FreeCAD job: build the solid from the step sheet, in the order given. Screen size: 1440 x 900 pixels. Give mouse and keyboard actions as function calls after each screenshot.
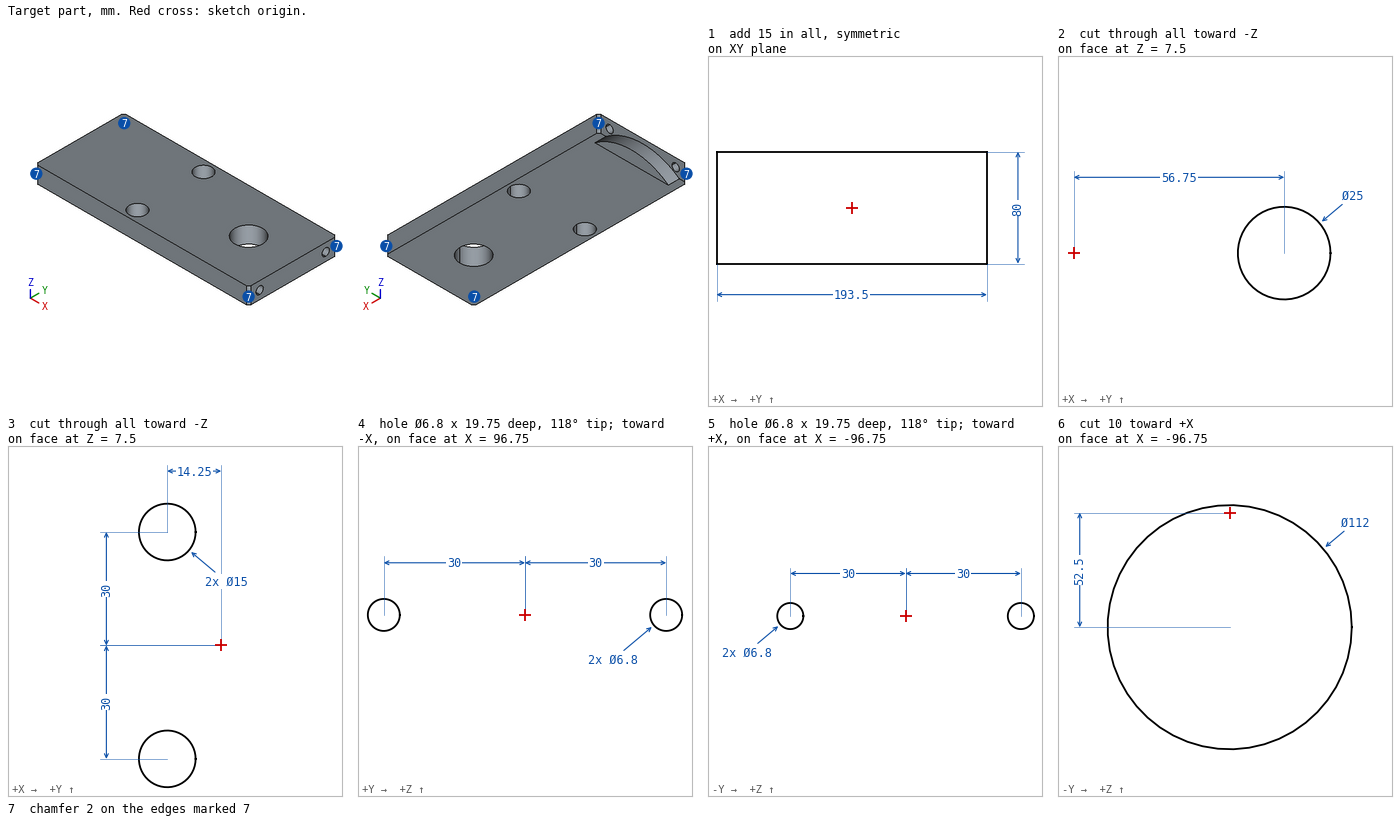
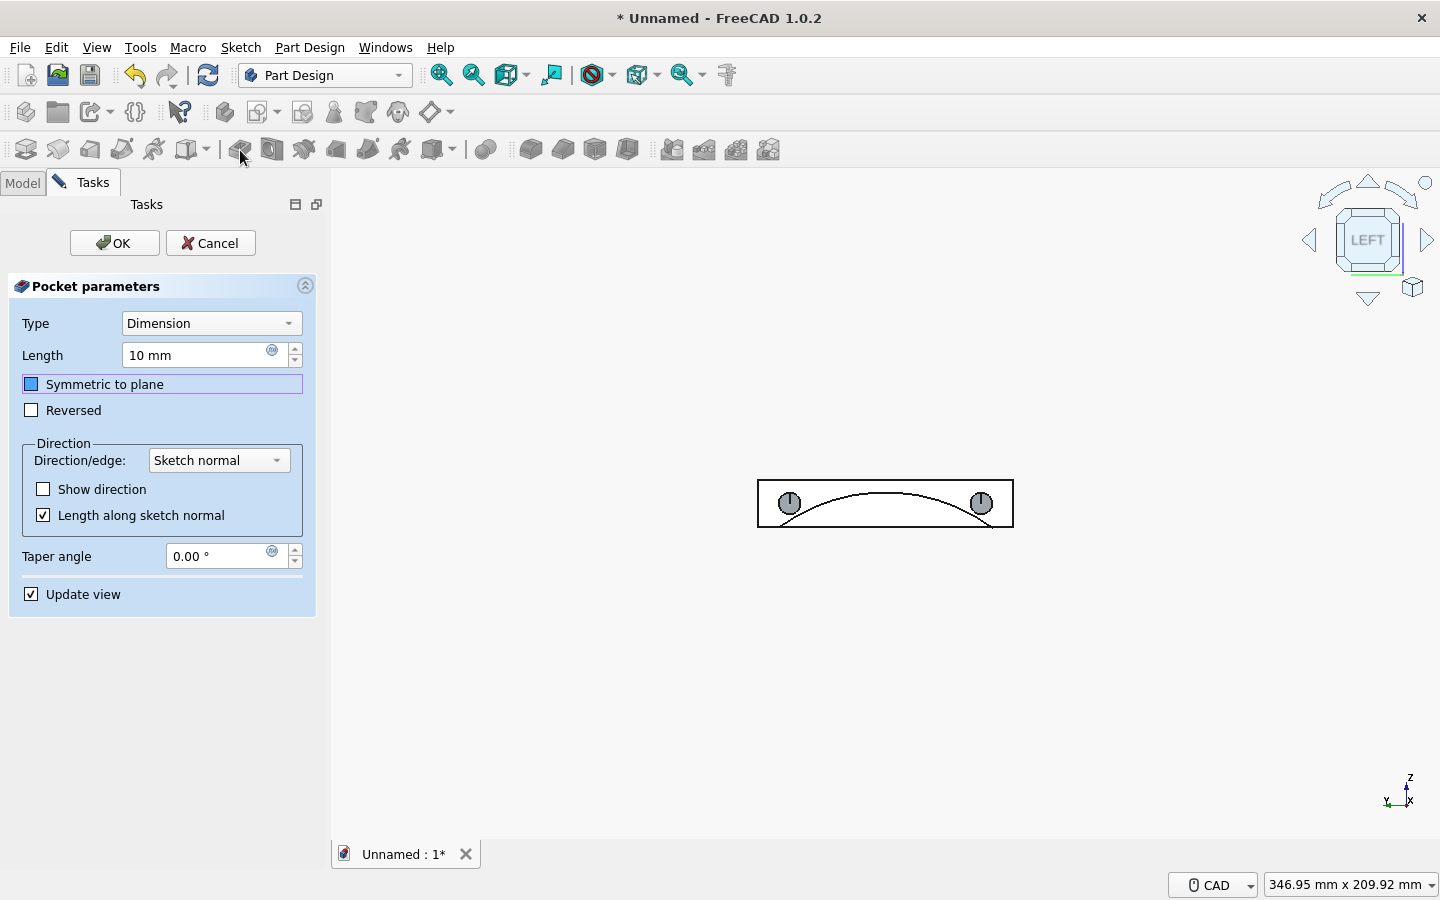
click(115, 243)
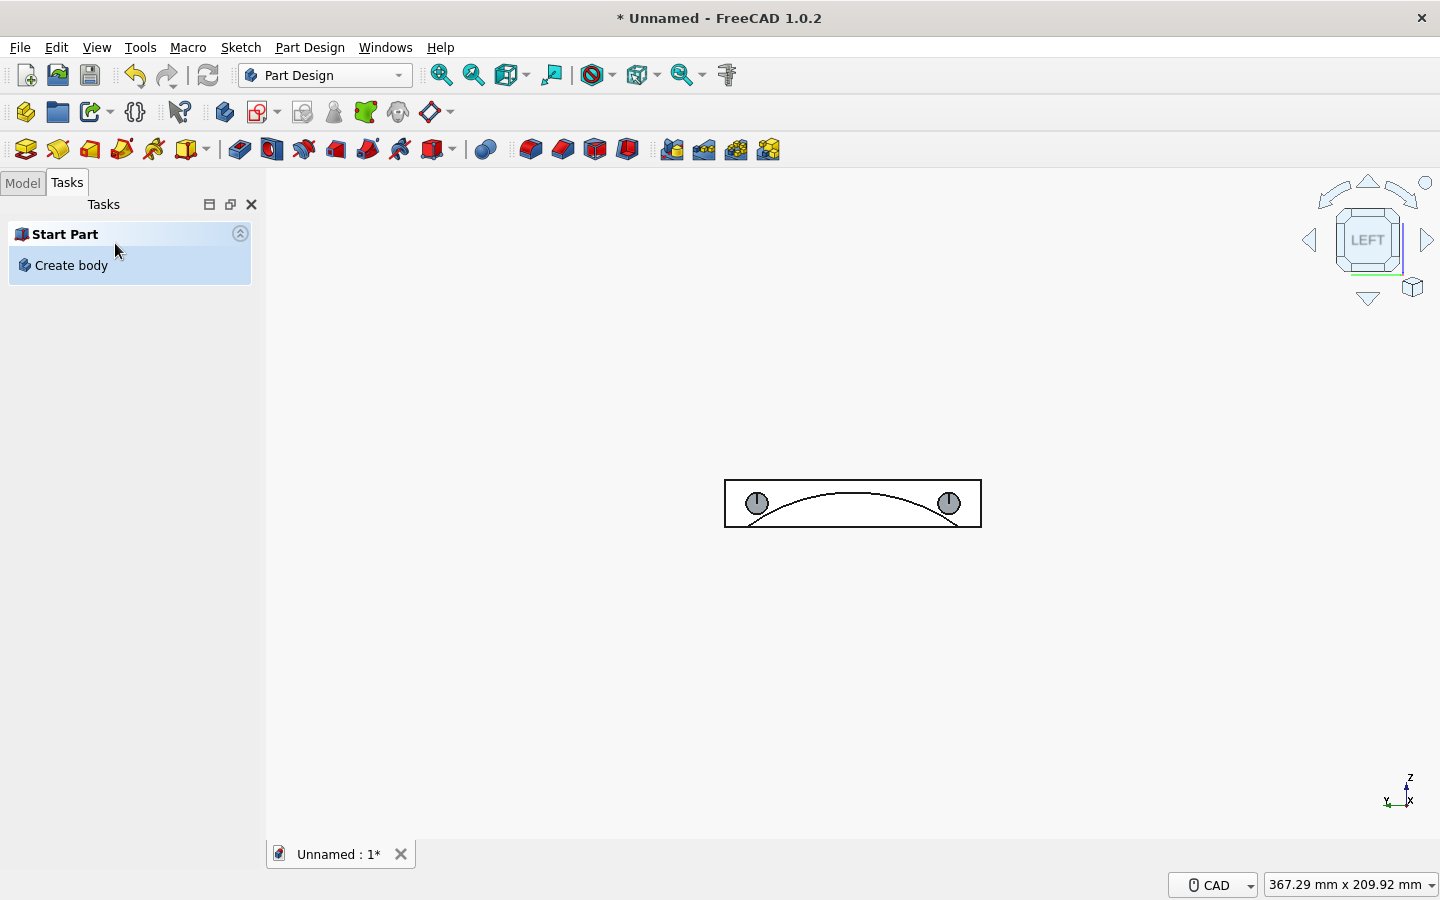
click(442, 76)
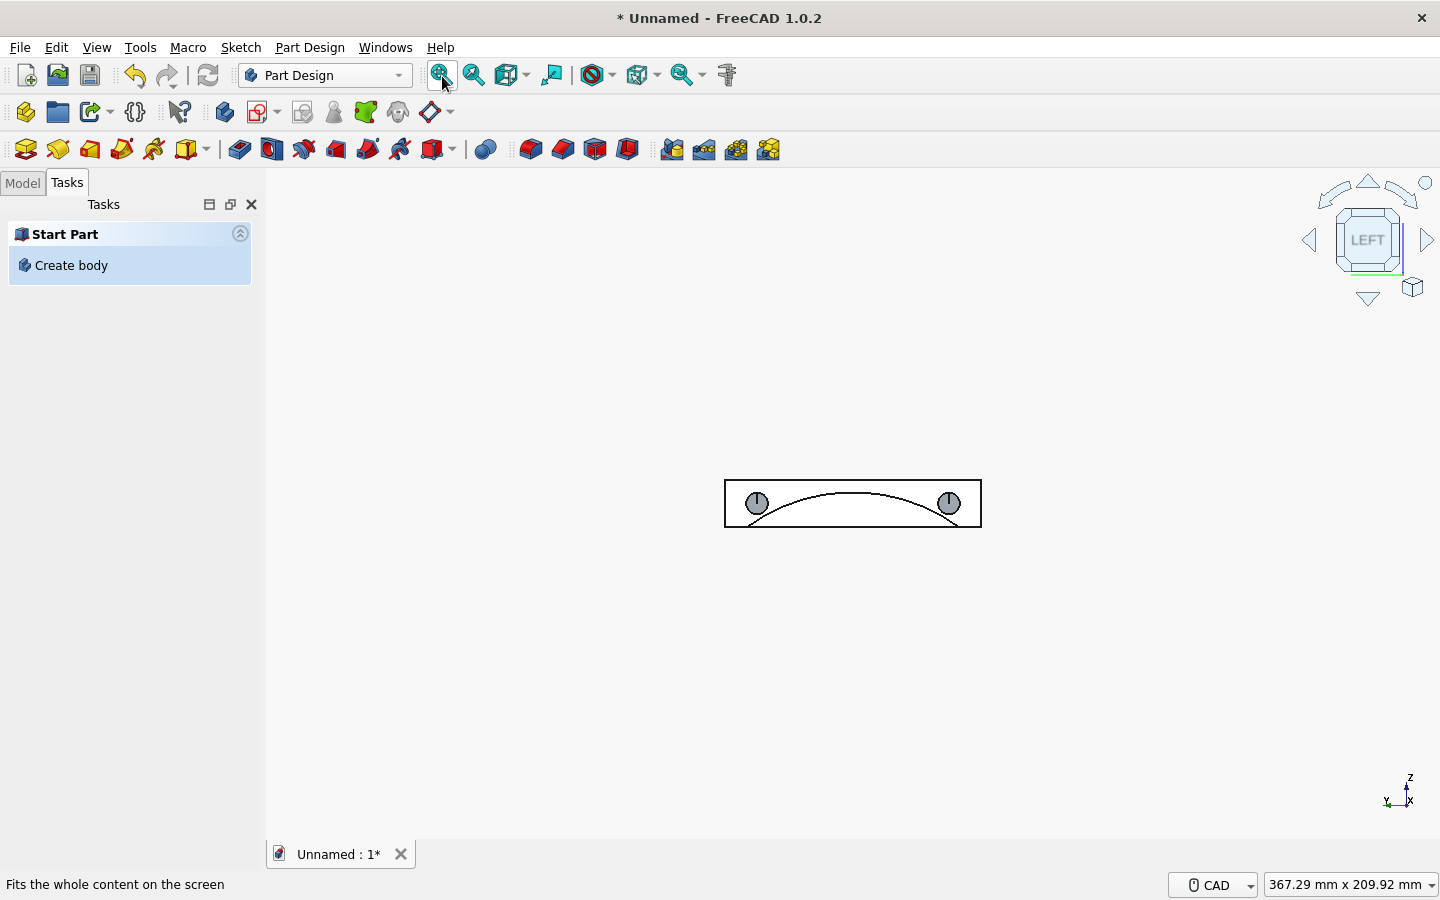
click(981, 502)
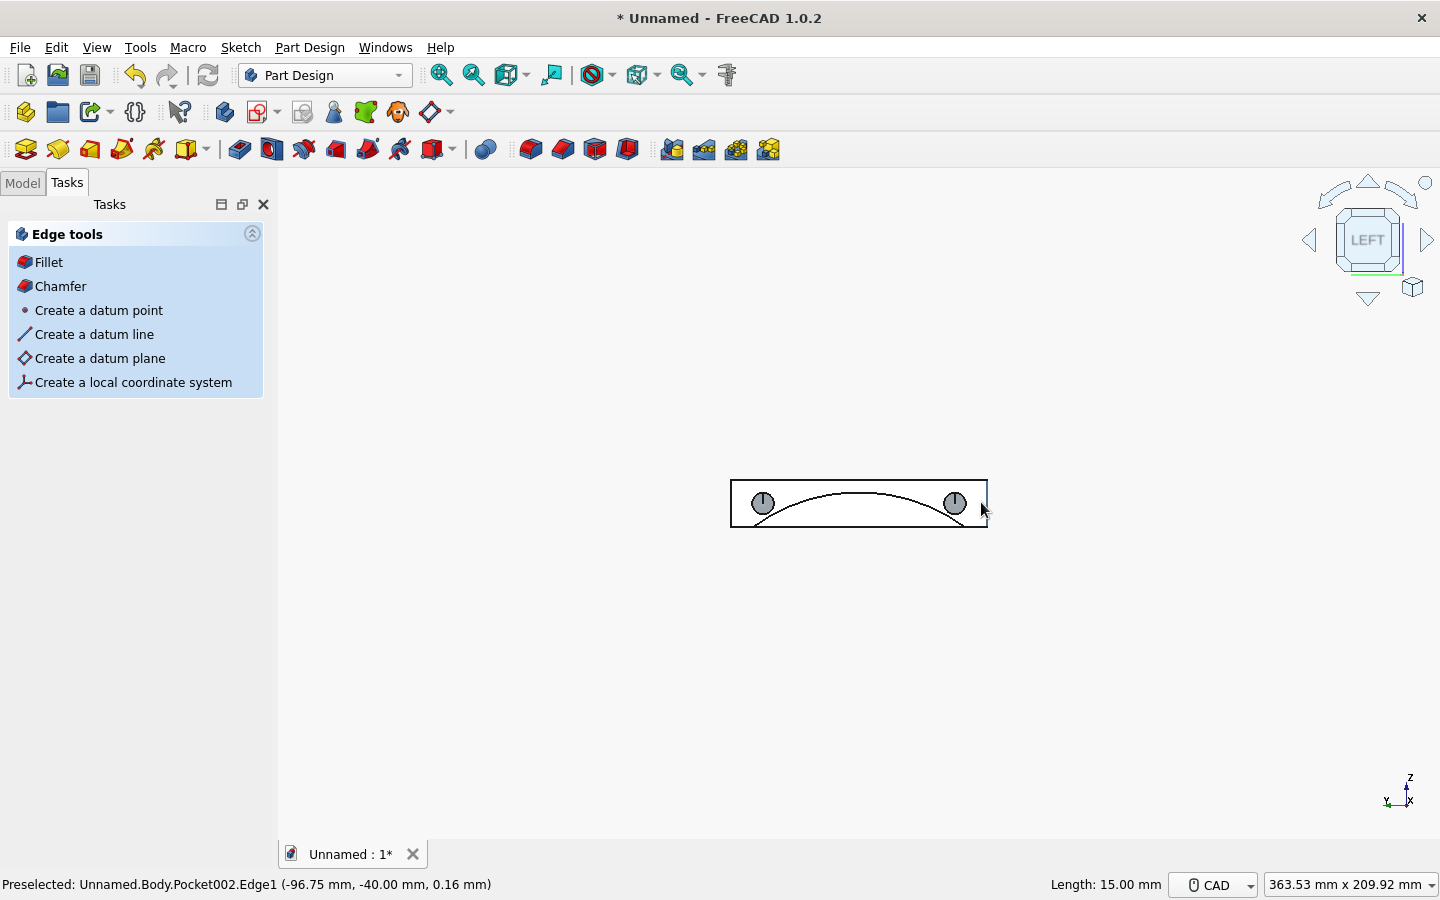
click(731, 502, ctrl)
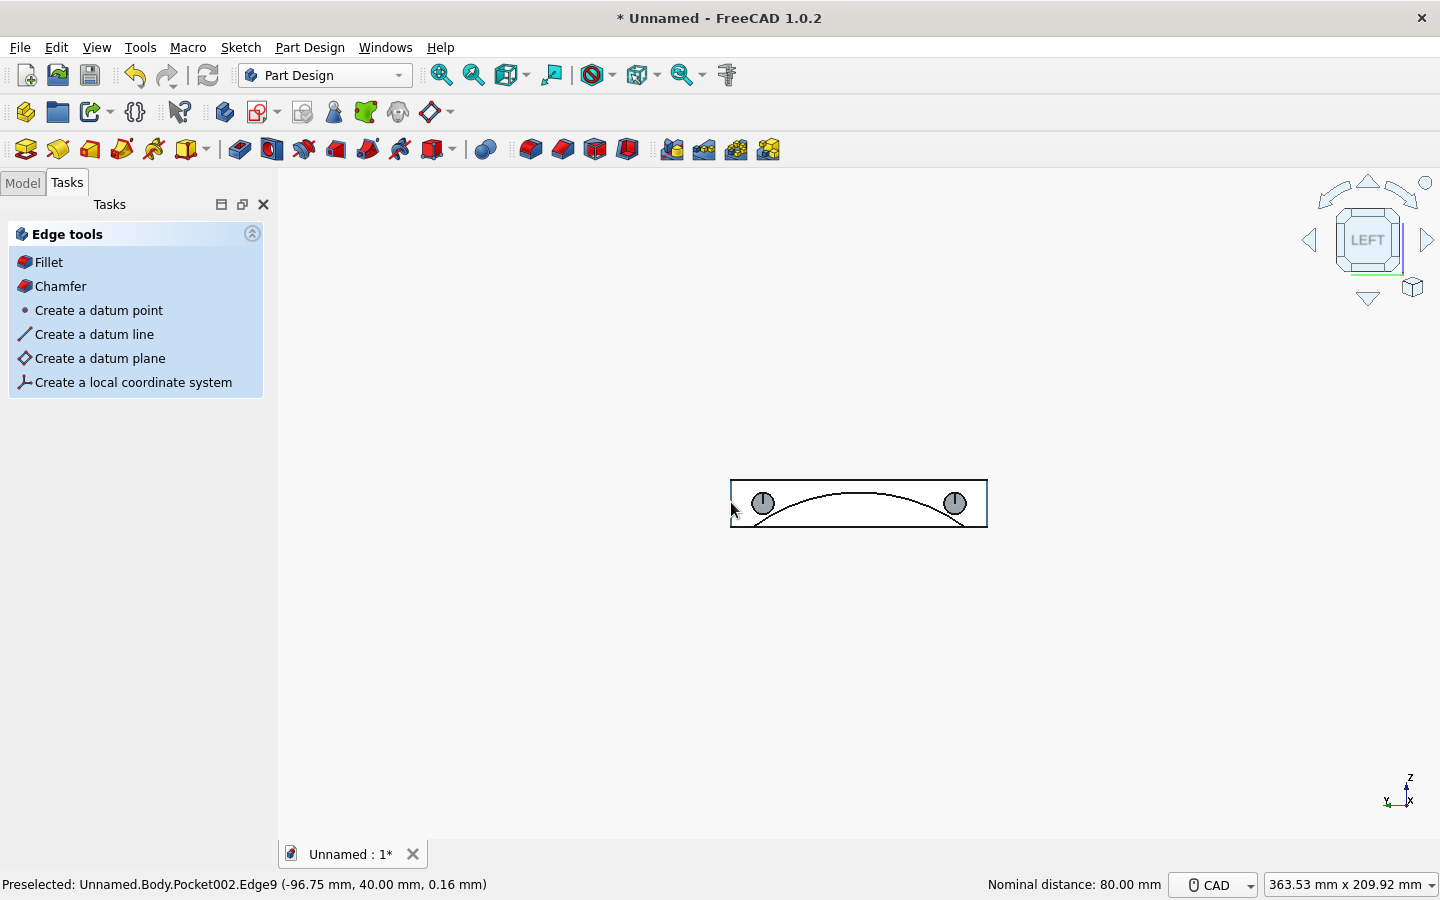
key(0)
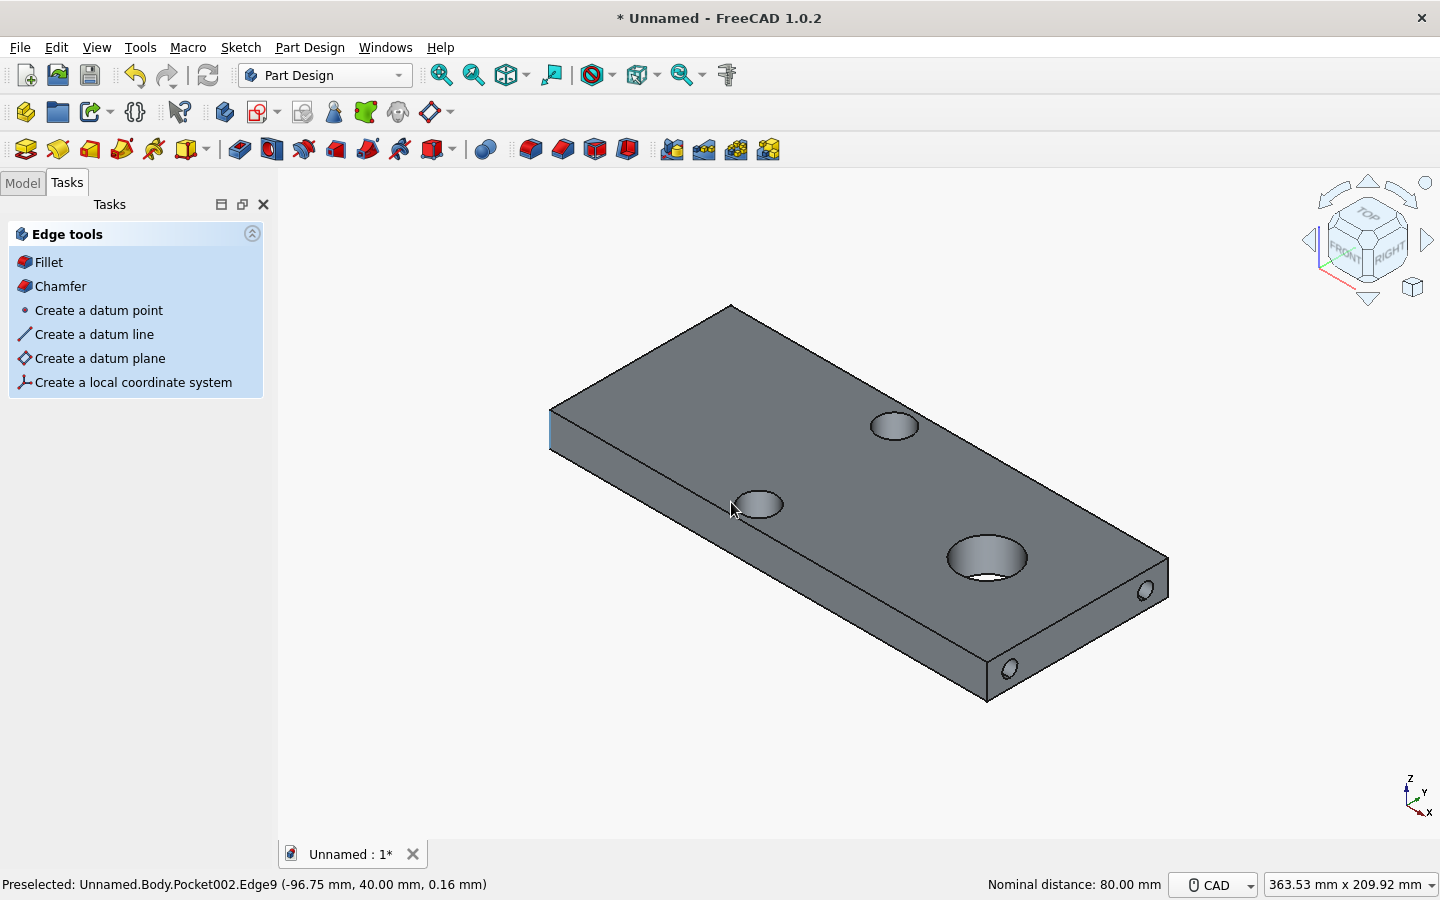
click(987, 681, ctrl)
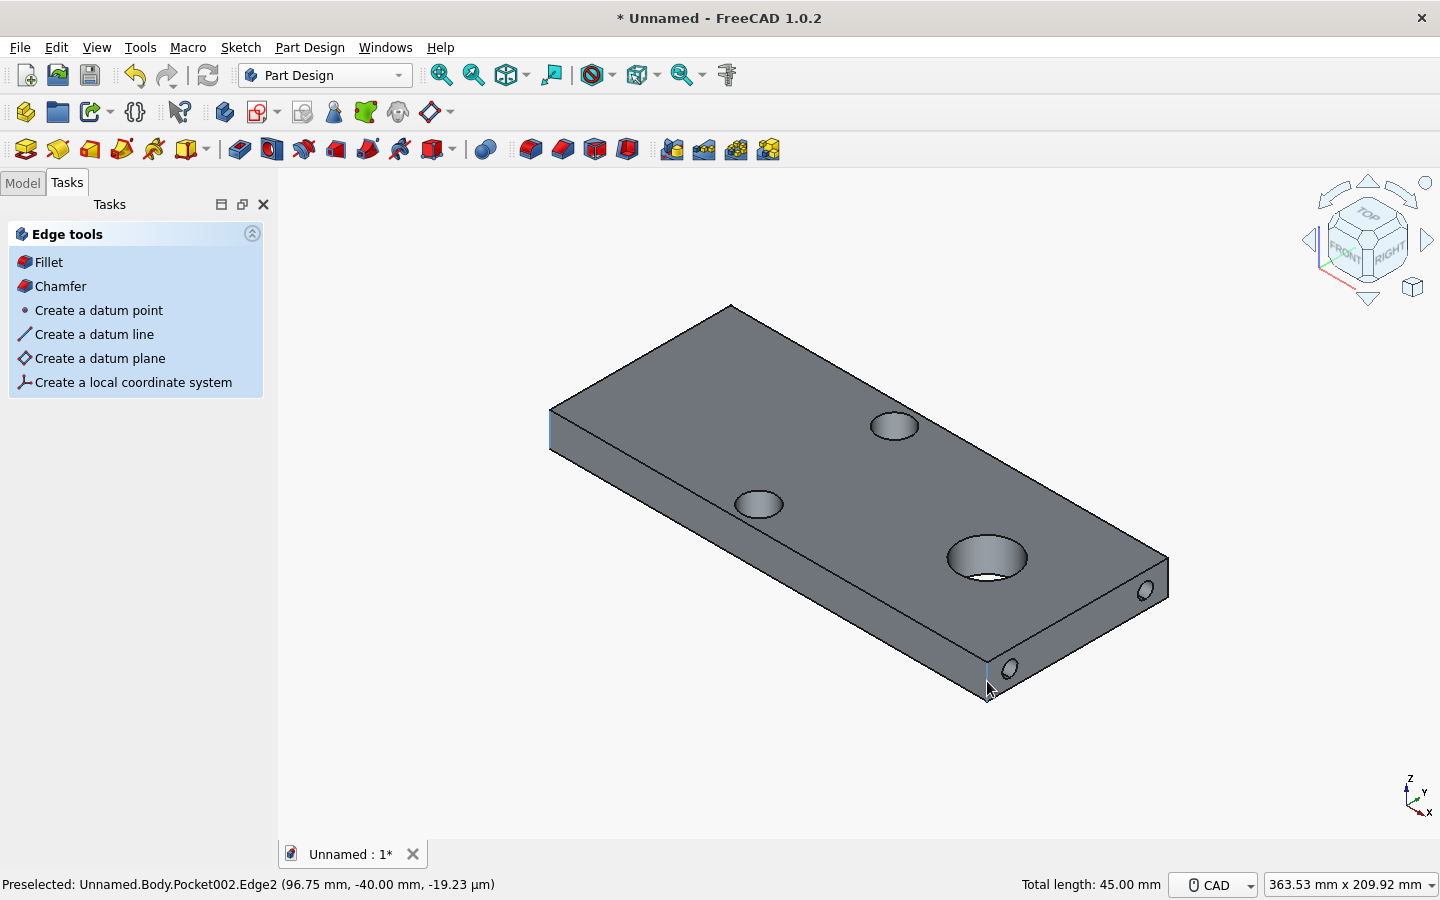
key(2)